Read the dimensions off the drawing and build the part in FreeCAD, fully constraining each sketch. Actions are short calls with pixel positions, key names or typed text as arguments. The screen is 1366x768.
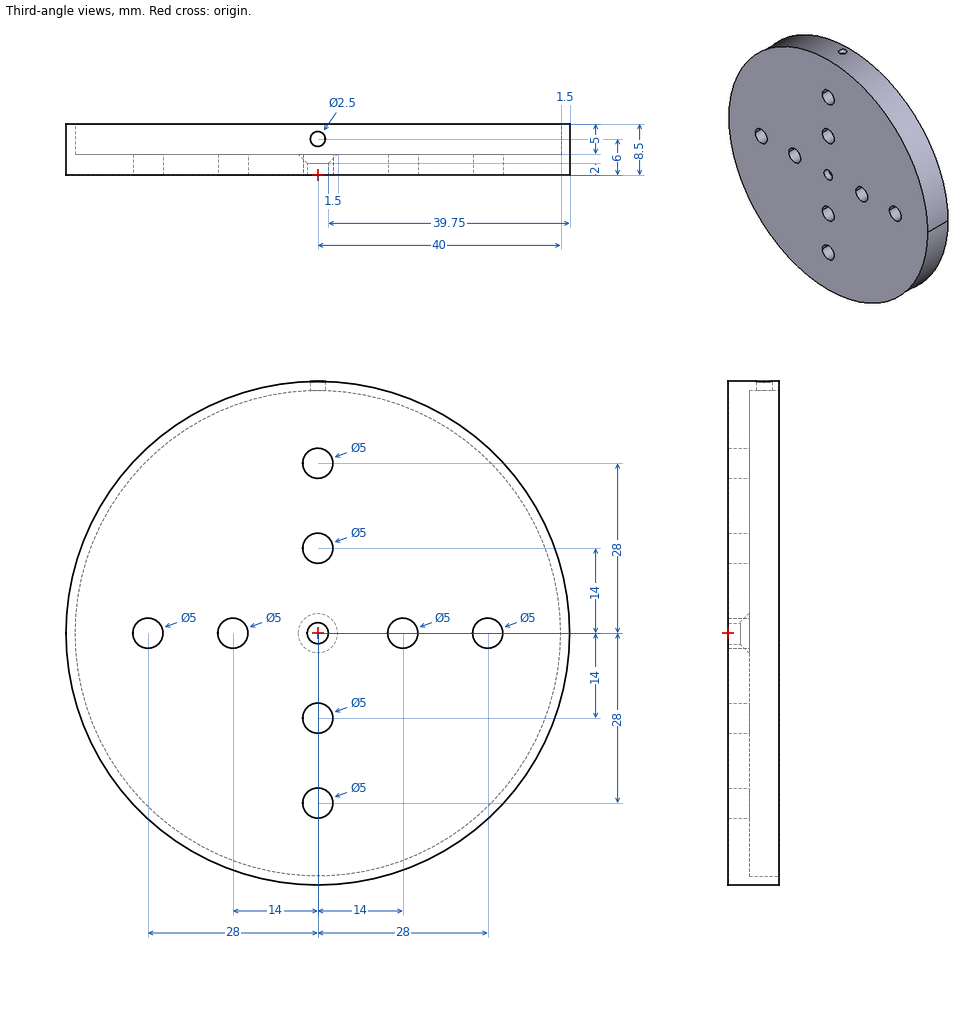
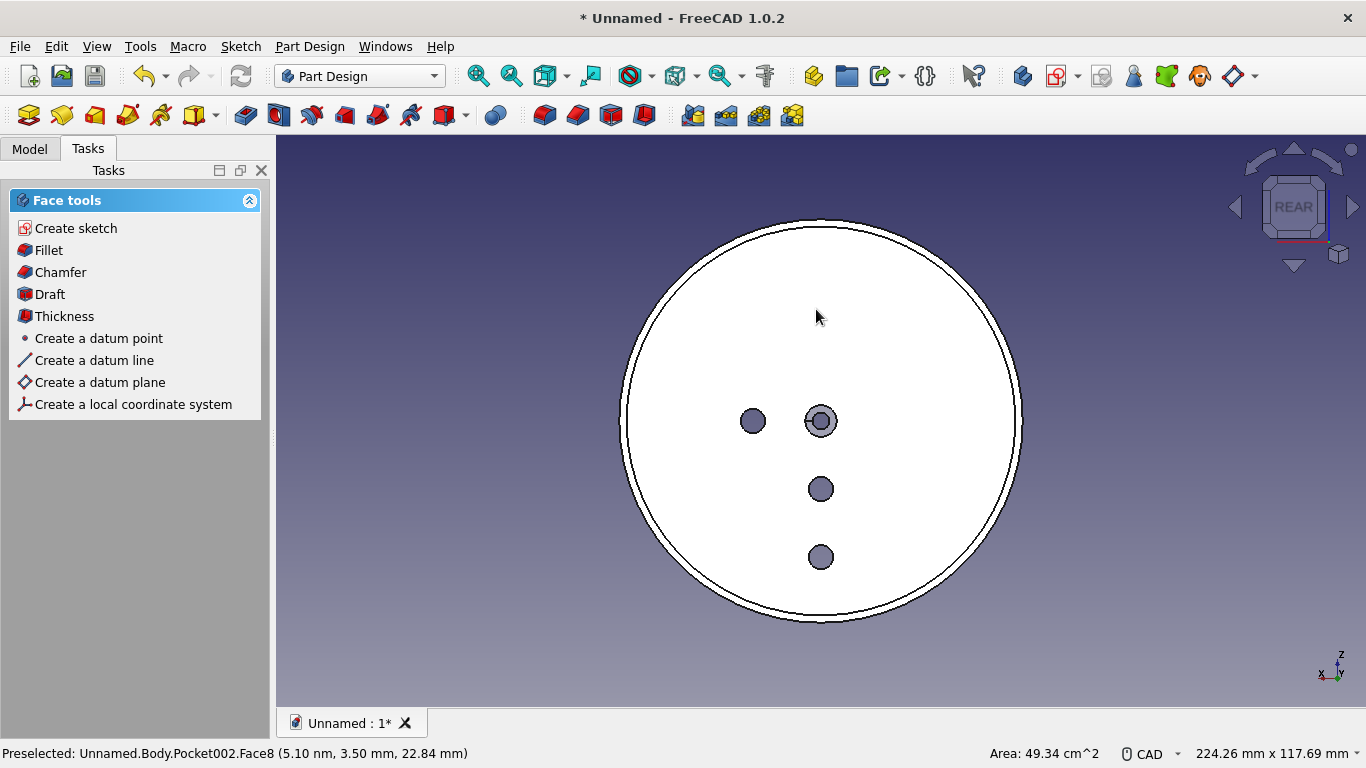
click(1056, 76)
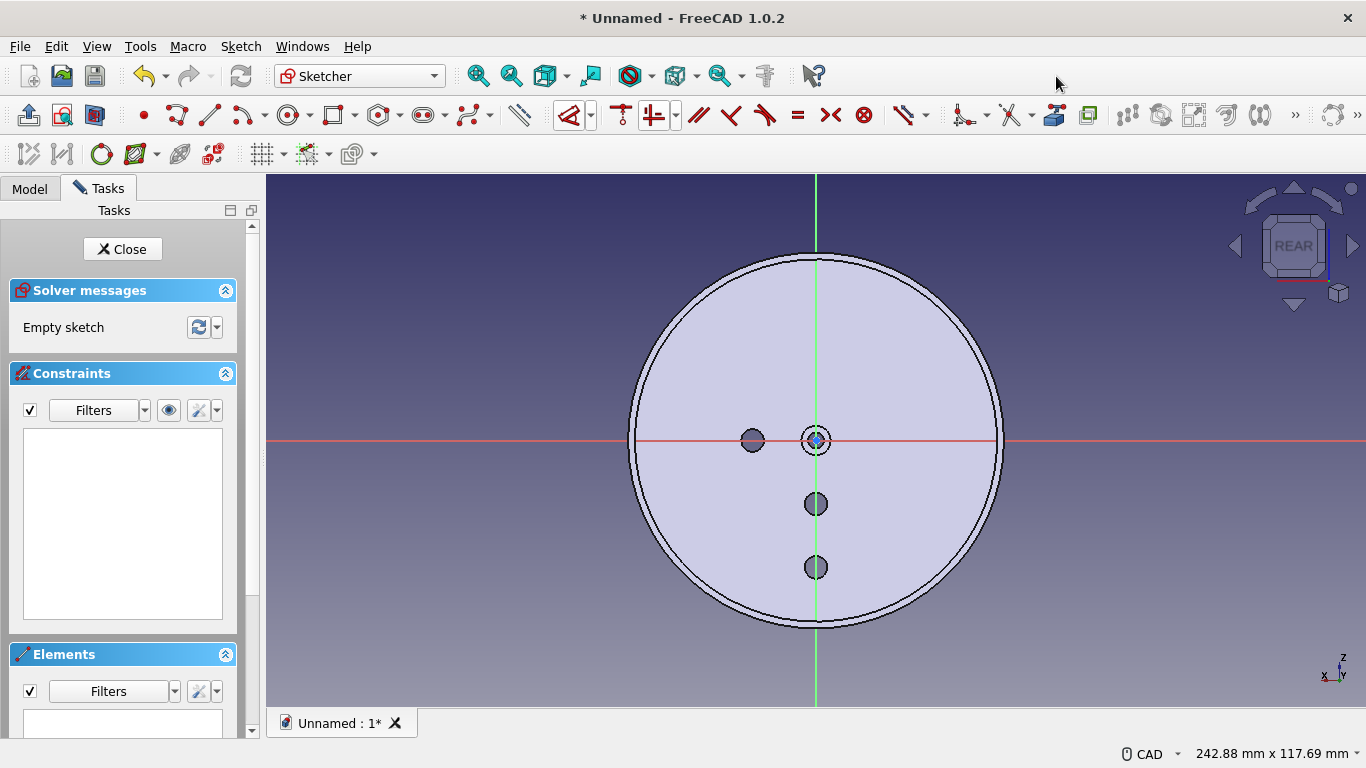
click(95, 116)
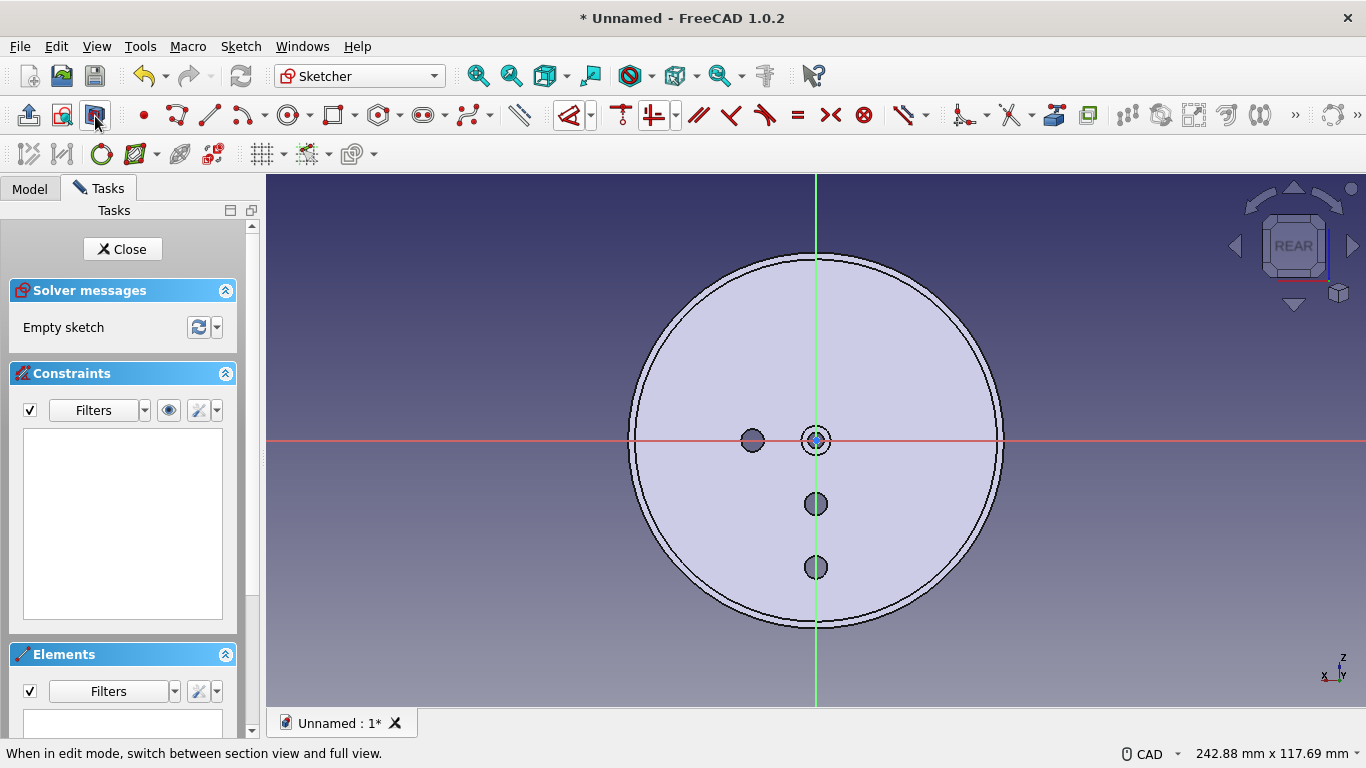
scroll(685, 441, up, 13)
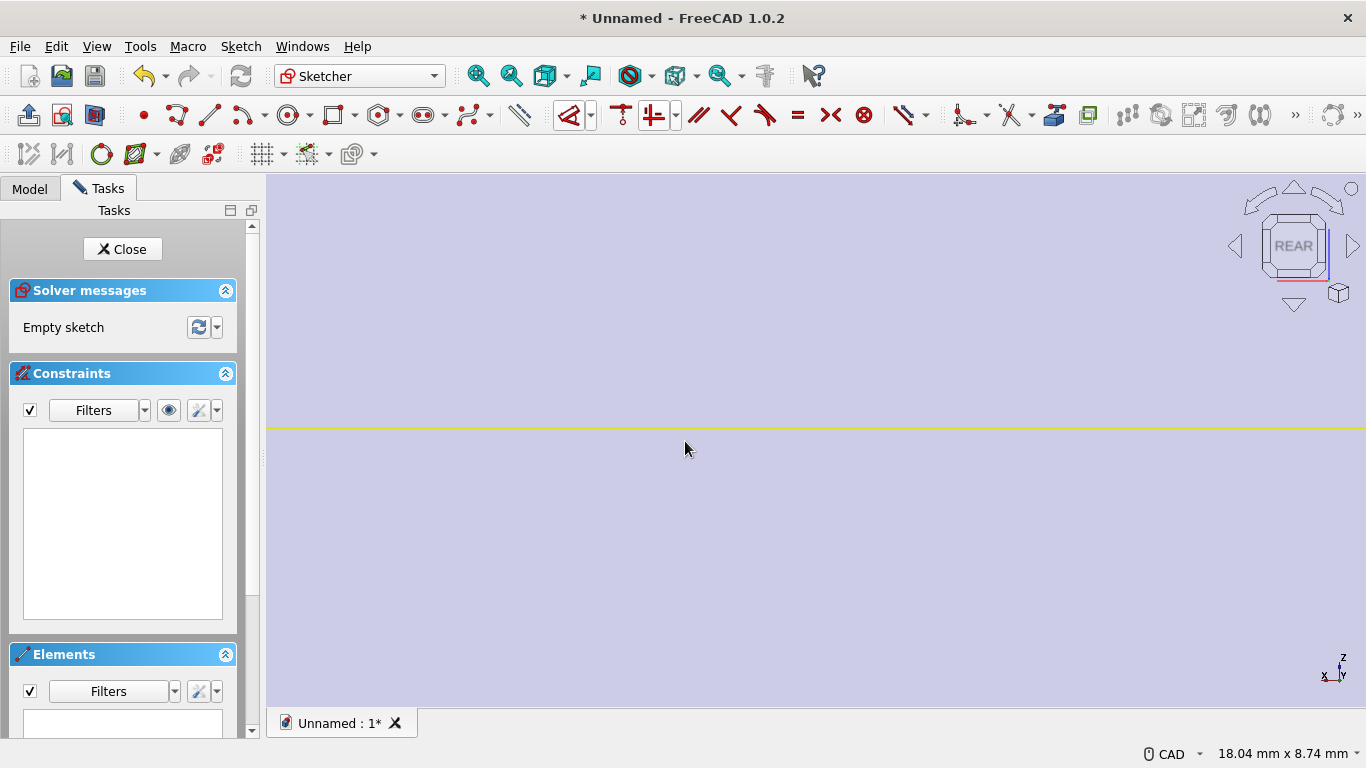
click(288, 116)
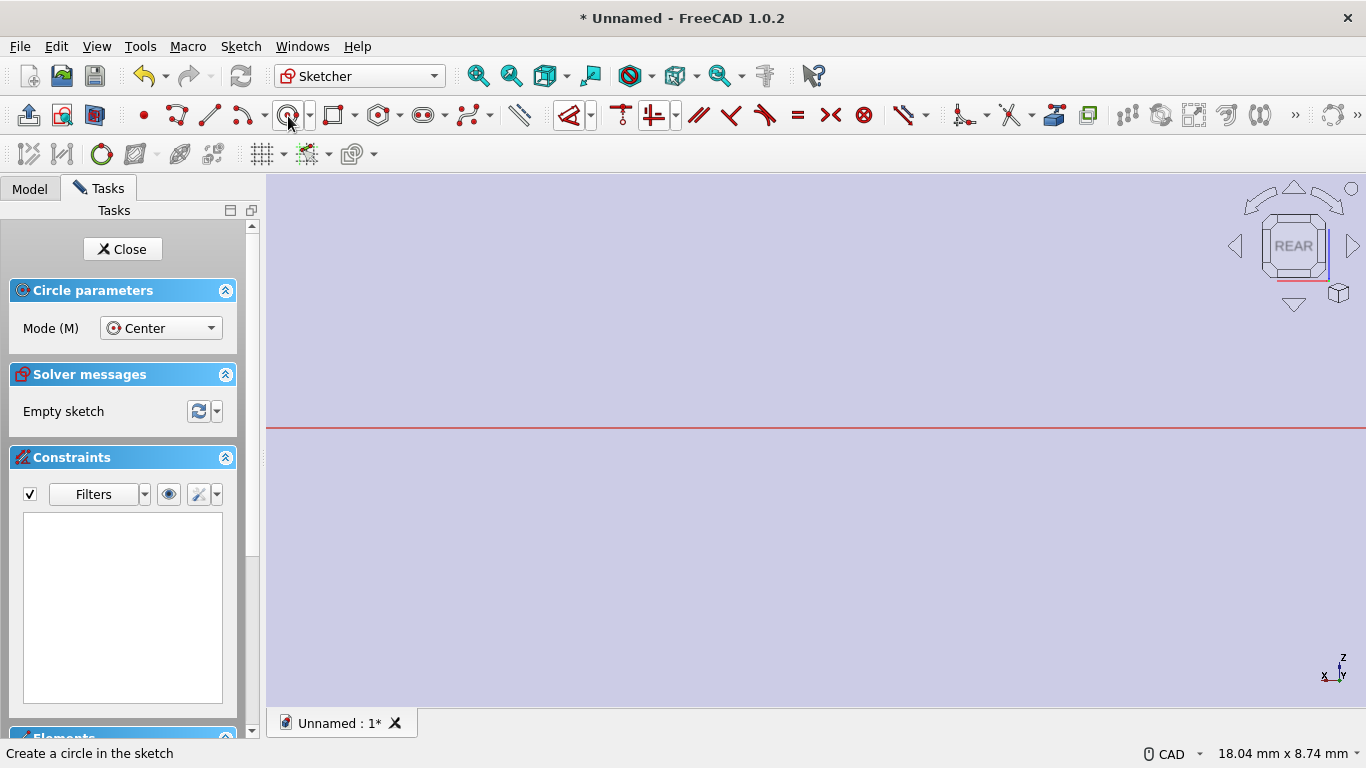
click(737, 428)
click(844, 320)
key(Escape)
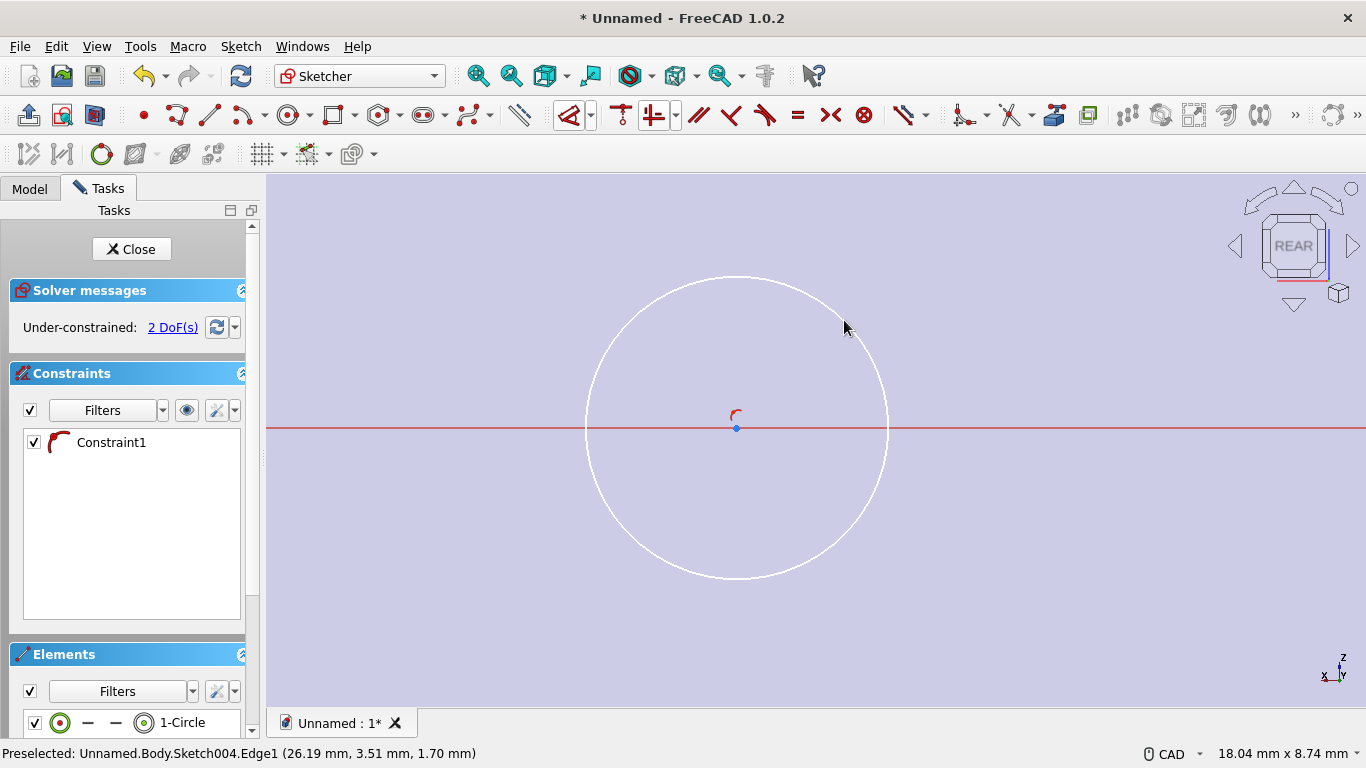
click(844, 321)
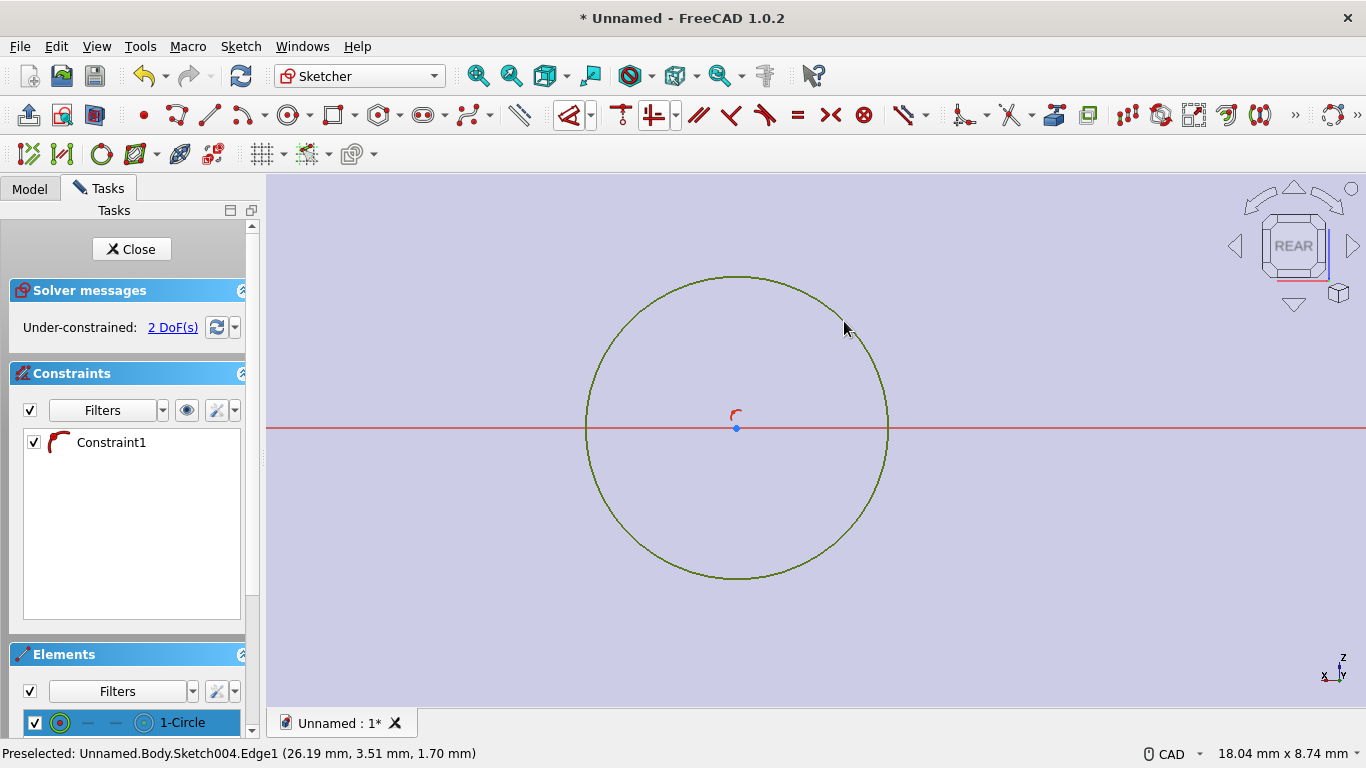
click(590, 116)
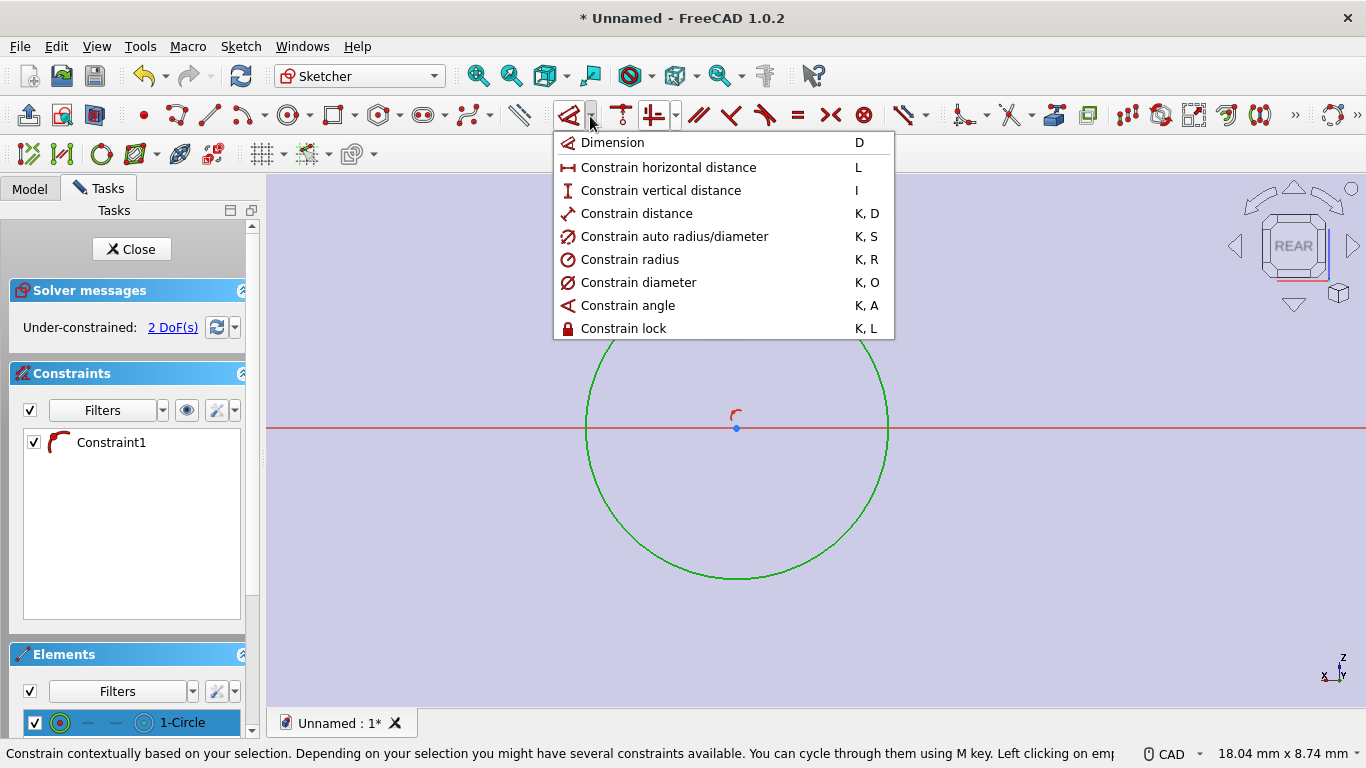
click(724, 282)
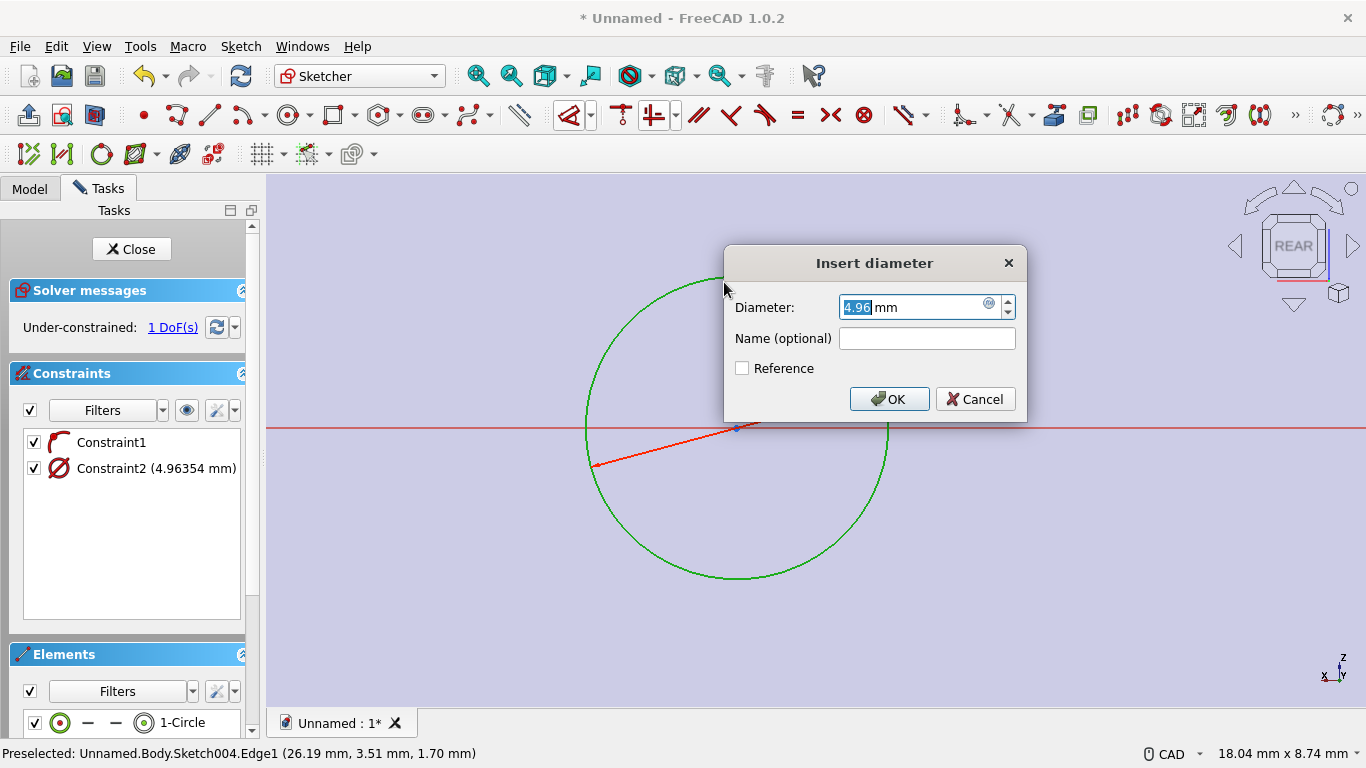
text(5)
key(Return)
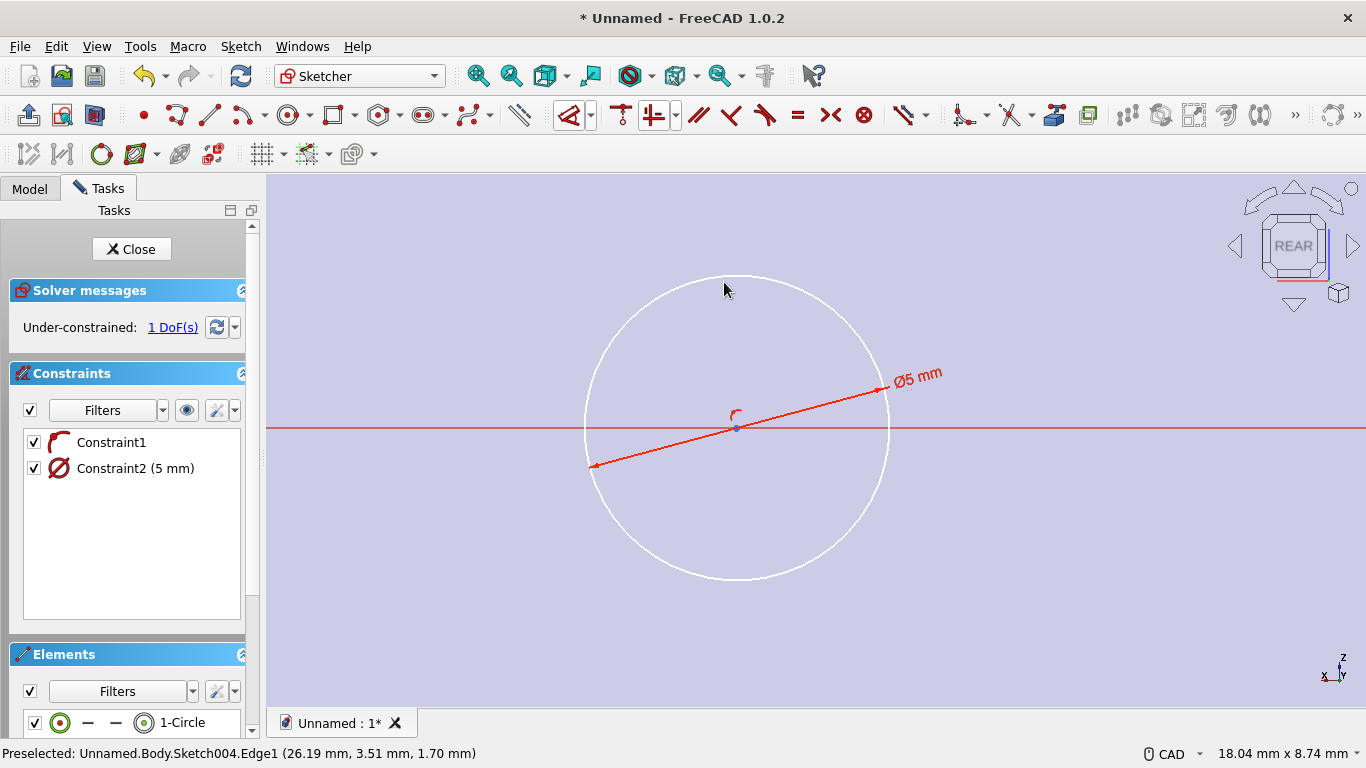
click(737, 428)